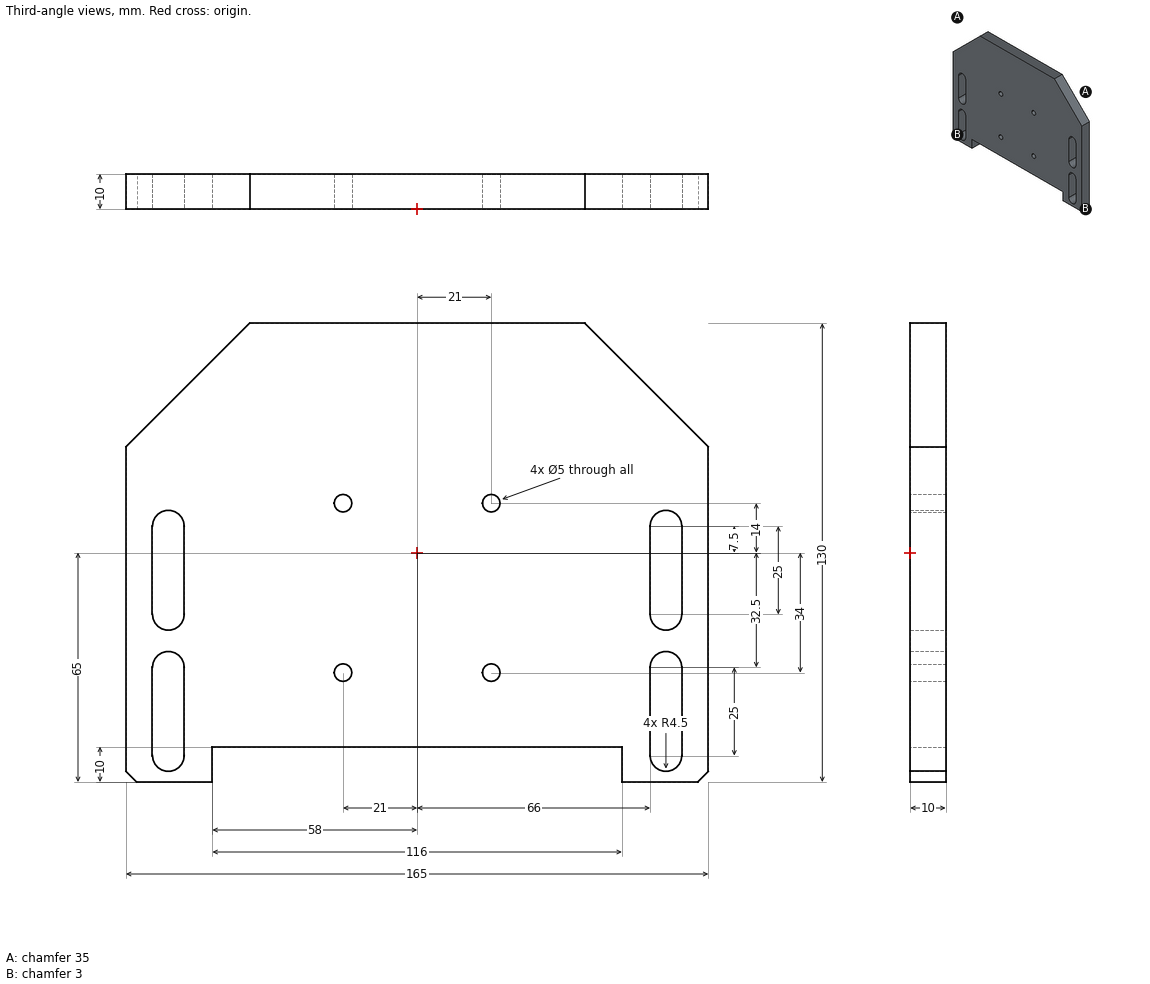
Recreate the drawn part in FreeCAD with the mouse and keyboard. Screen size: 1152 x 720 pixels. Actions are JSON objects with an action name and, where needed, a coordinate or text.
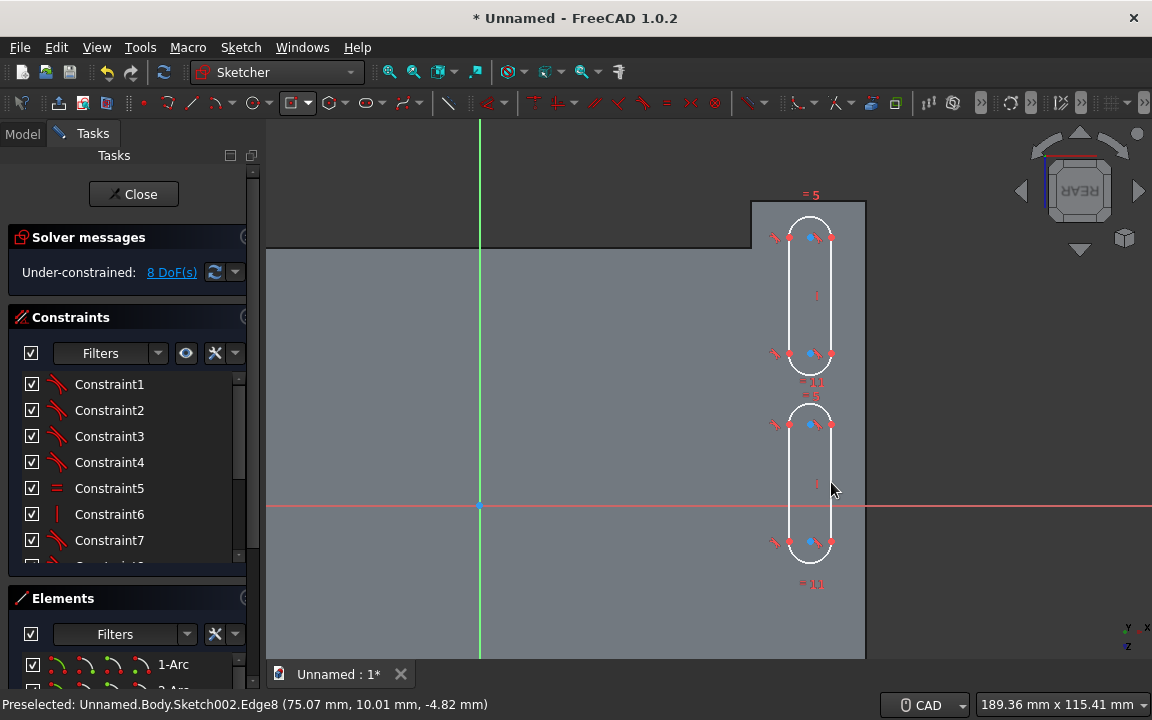
{"action": "left_click", "coordinate": [798, 371]}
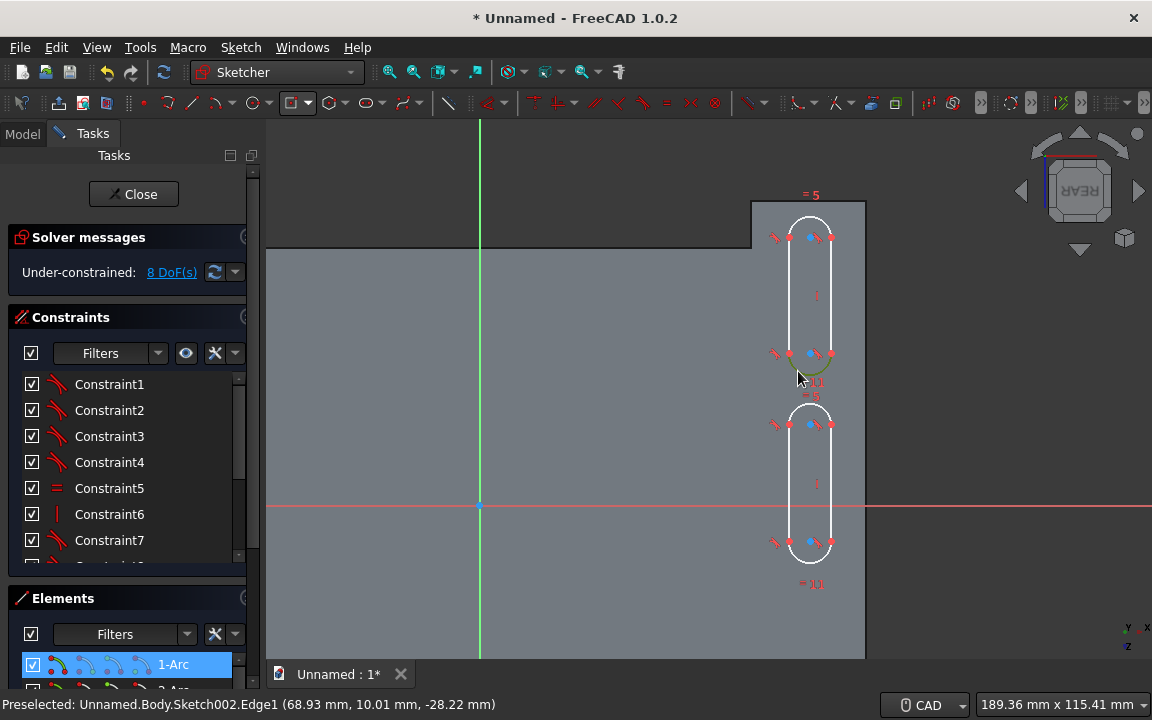
{"action": "left_click", "coordinate": [798, 559]}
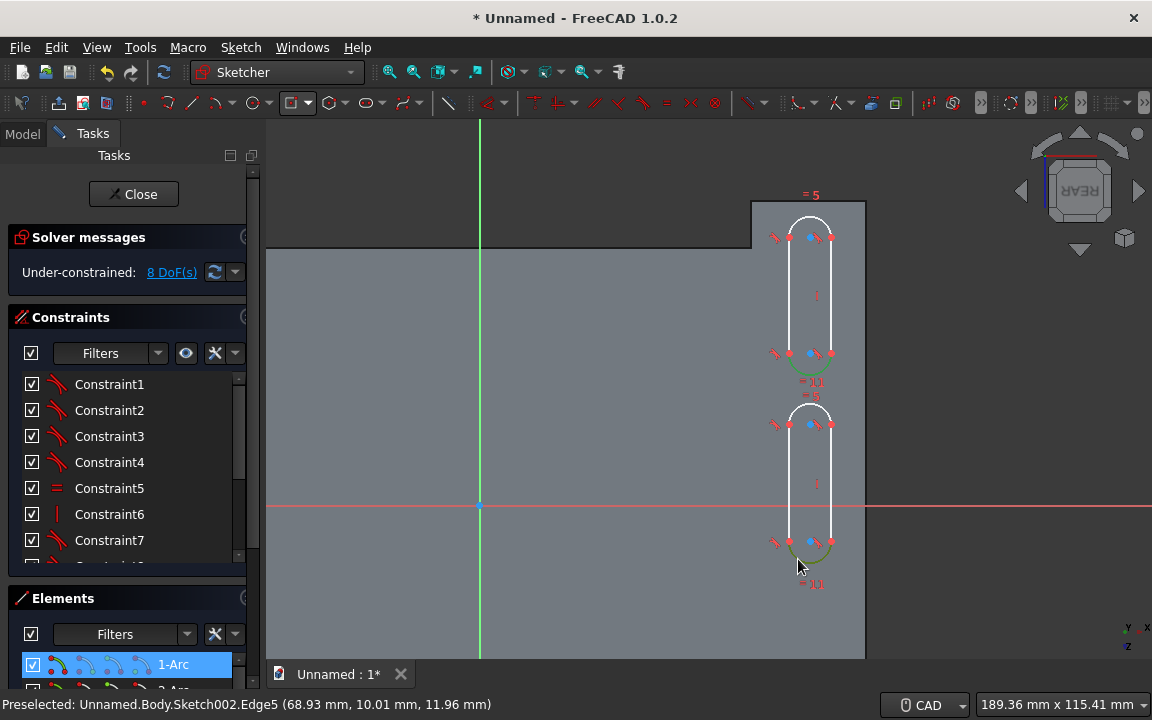
{"action": "left_click", "coordinate": [668, 104]}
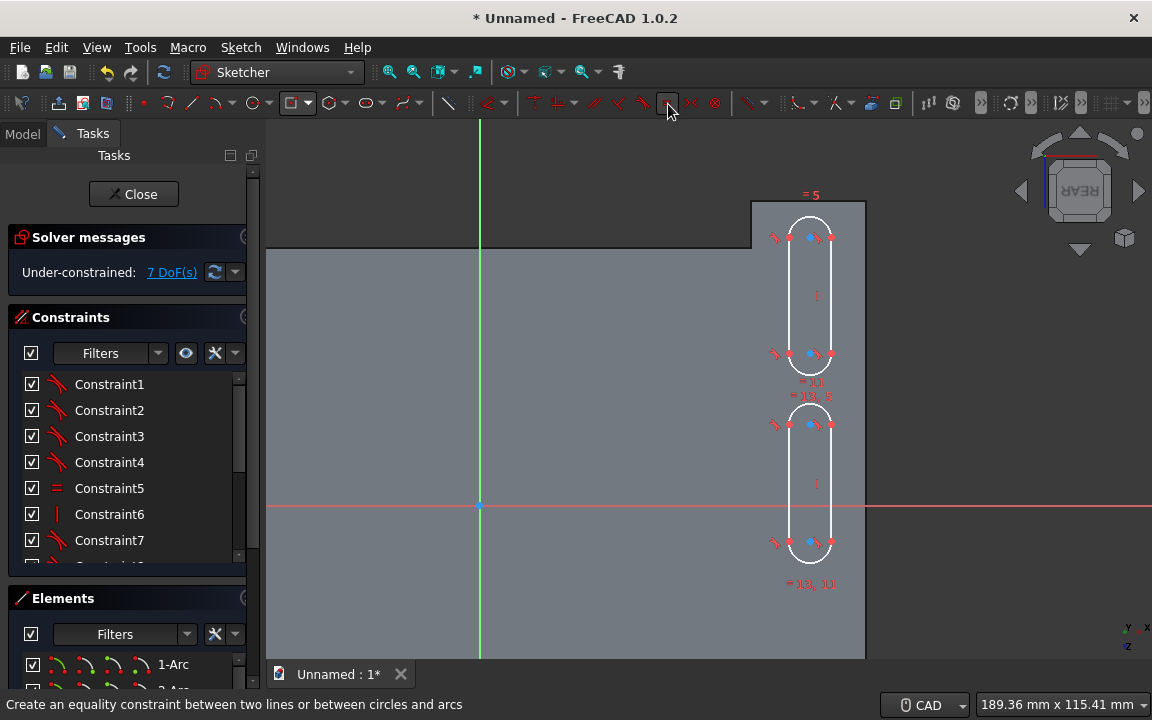
{"action": "key", "text": "d"}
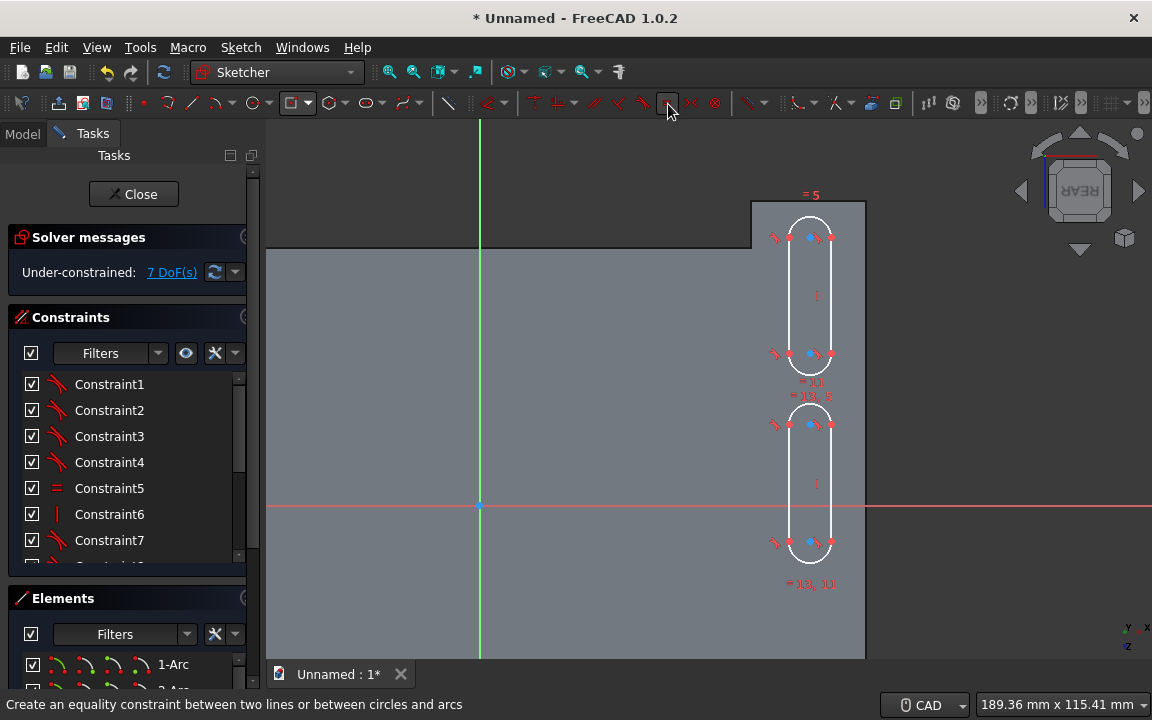
{"action": "scroll", "coordinate": [798, 371], "scroll_direction": "up", "scroll_amount": 4}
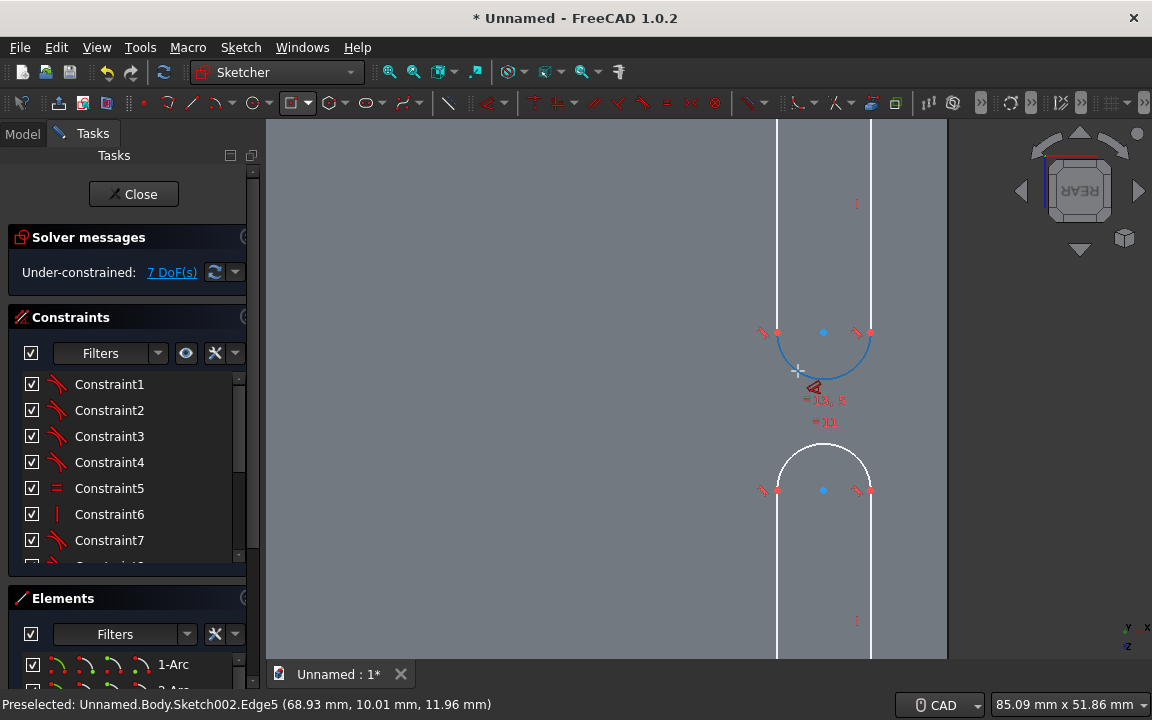
{"action": "left_click", "coordinate": [796, 370]}
{"action": "left_click", "coordinate": [777, 396]}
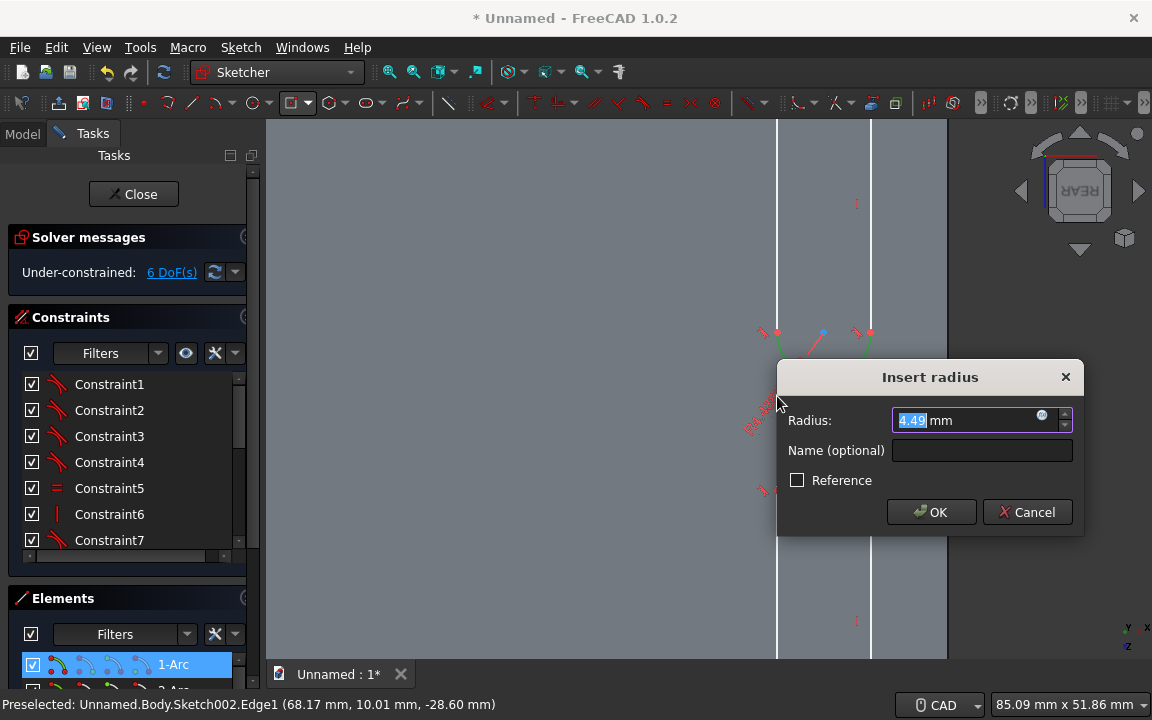
{"action": "type", "text": "4.5"}
{"action": "key", "text": "Return"}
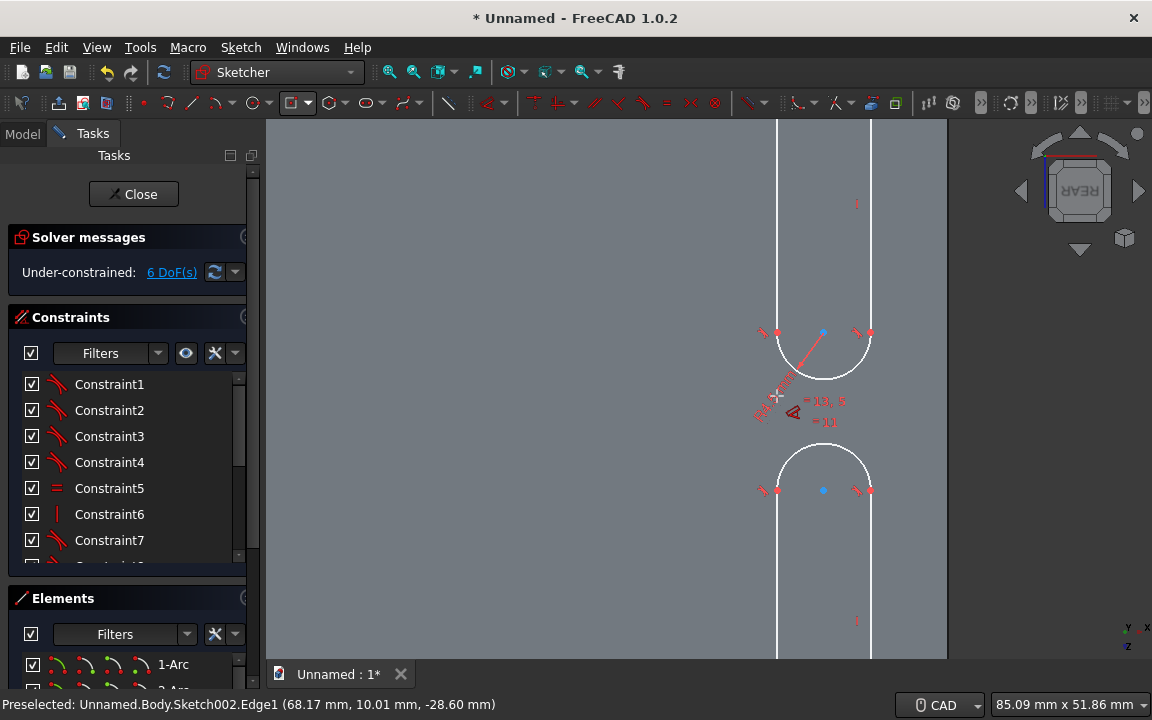
{"action": "left_click", "coordinate": [777, 255]}
{"action": "left_click", "coordinate": [811, 240]}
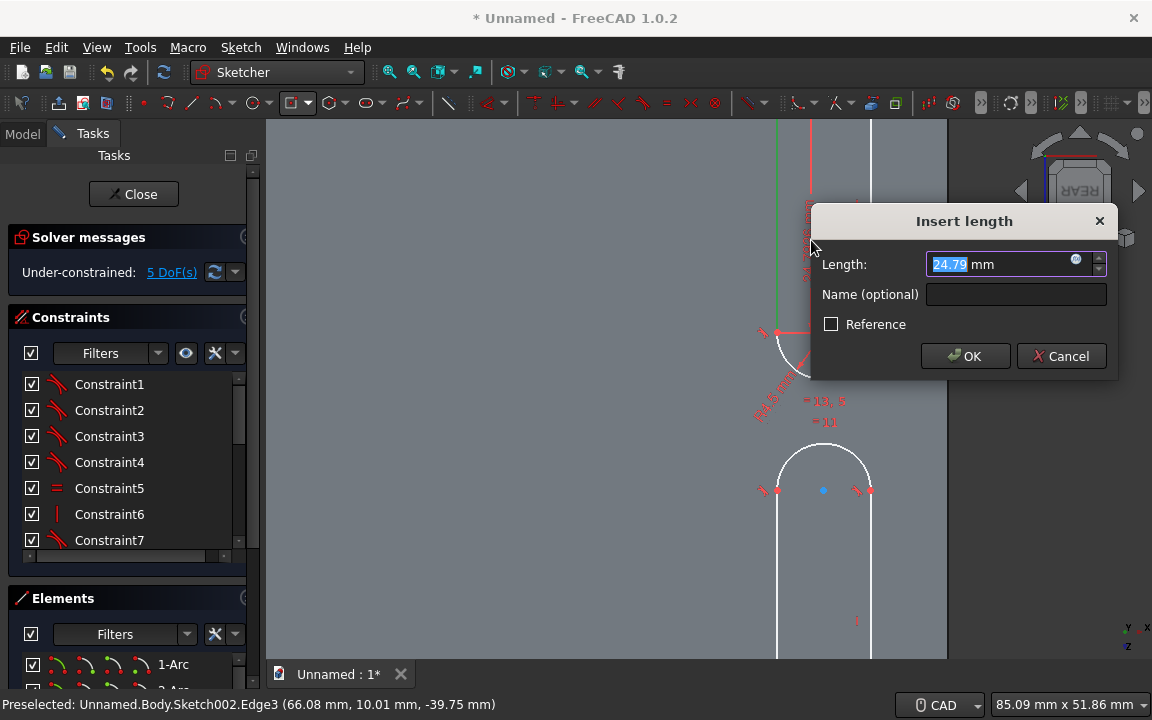
{"action": "type", "text": "25"}
{"action": "key", "text": "Return"}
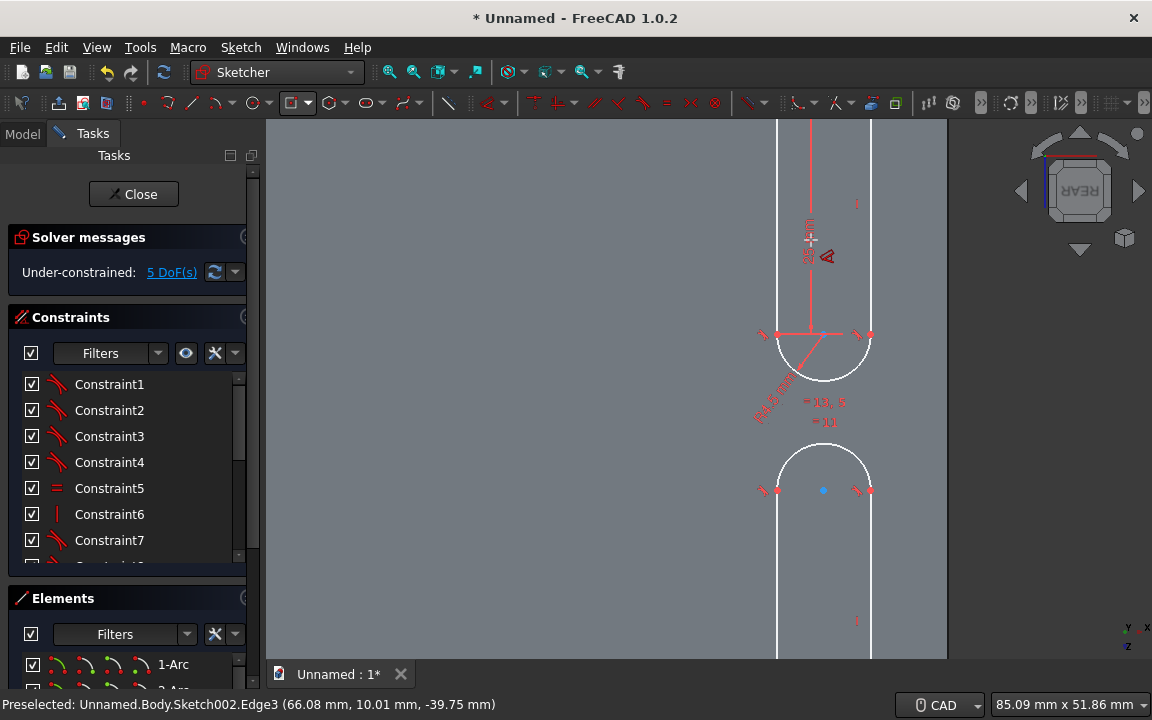
{"action": "left_click", "coordinate": [777, 569]}
{"action": "left_click", "coordinate": [811, 561]}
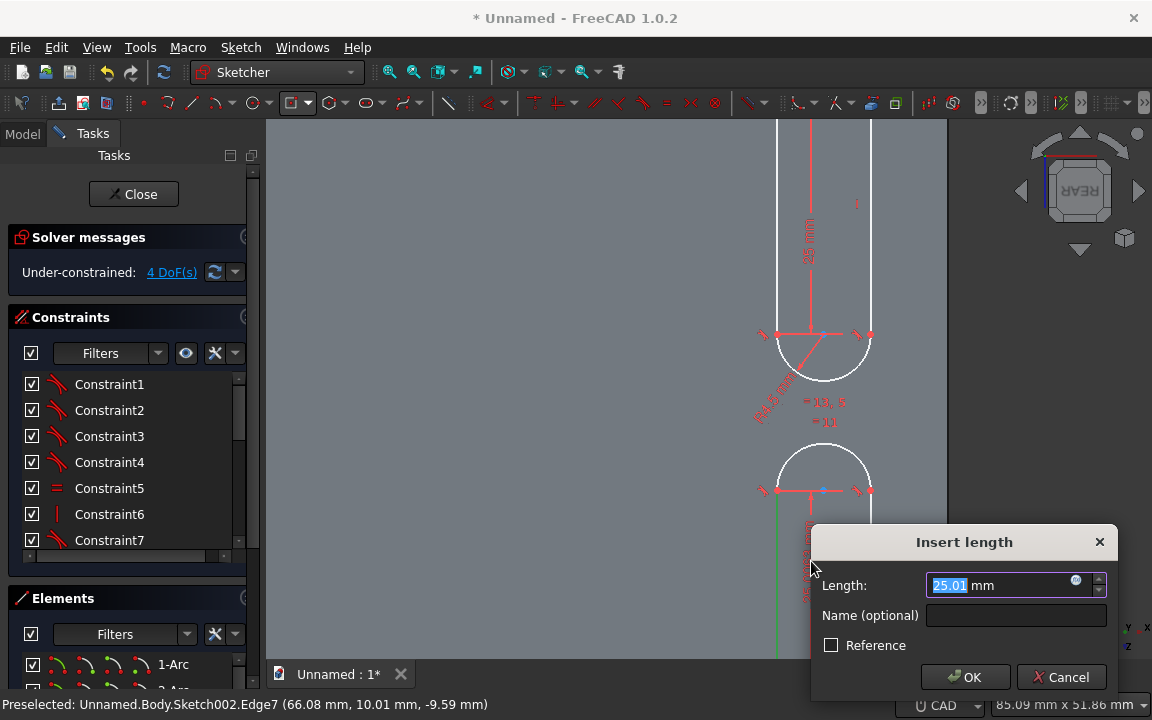
{"action": "type", "text": "25"}
{"action": "key", "text": "Return"}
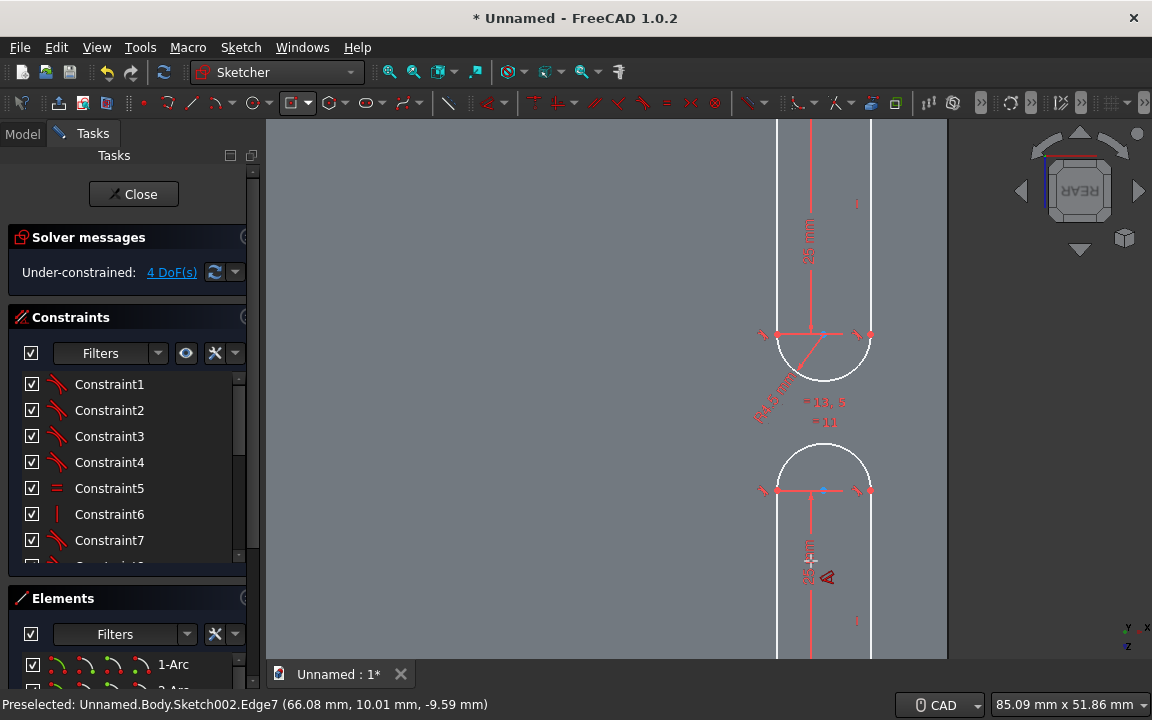
{"action": "left_click", "coordinate": [777, 334]}
{"action": "left_click", "coordinate": [536, 300]}